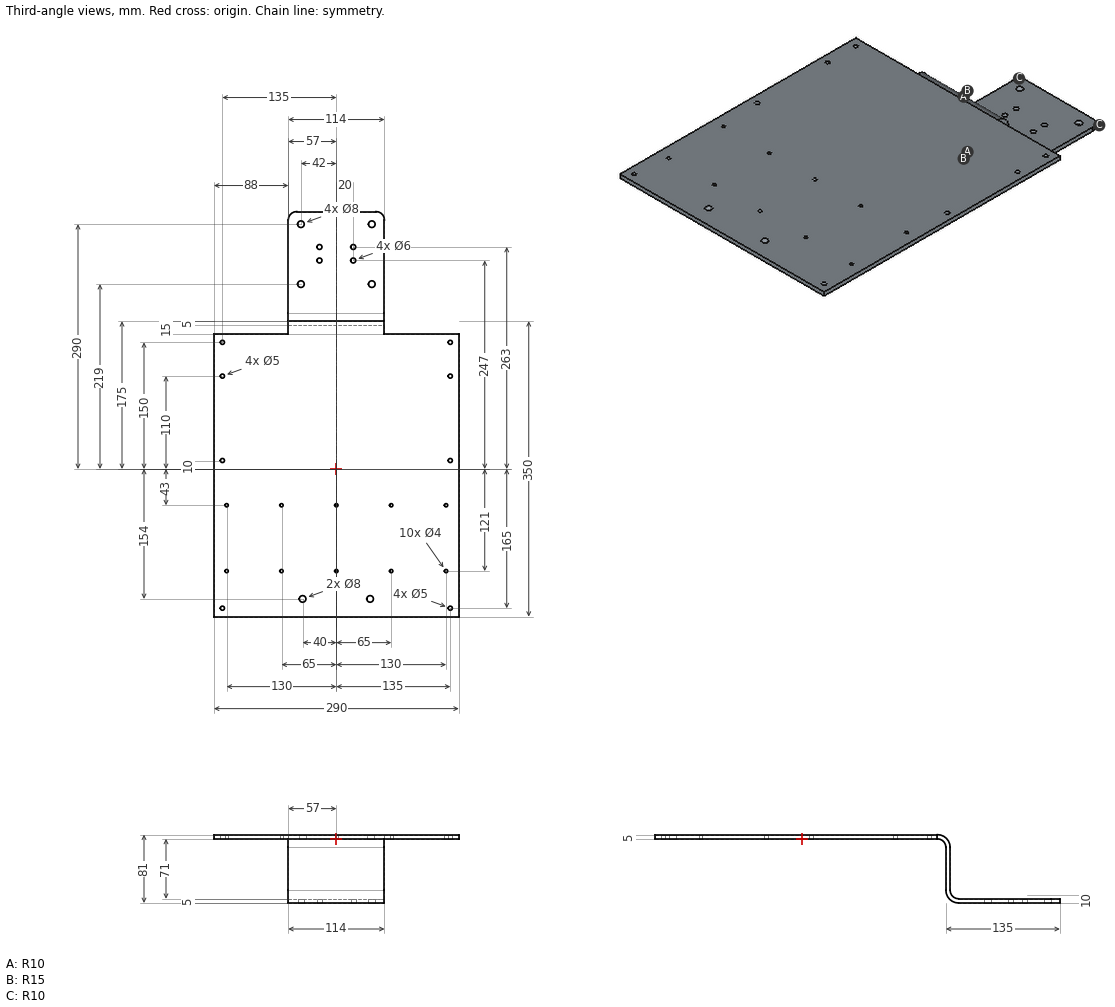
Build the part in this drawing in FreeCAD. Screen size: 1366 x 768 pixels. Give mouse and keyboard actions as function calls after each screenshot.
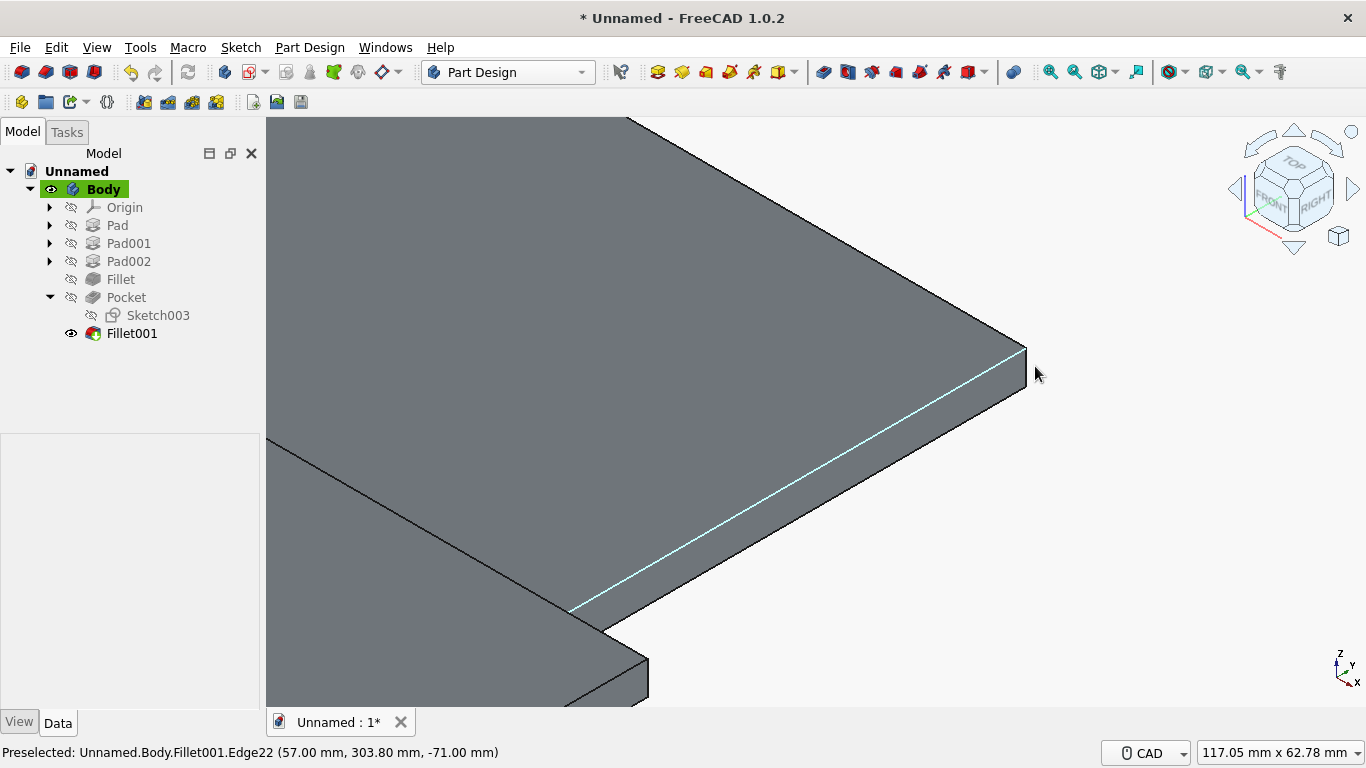
click(1052, 72)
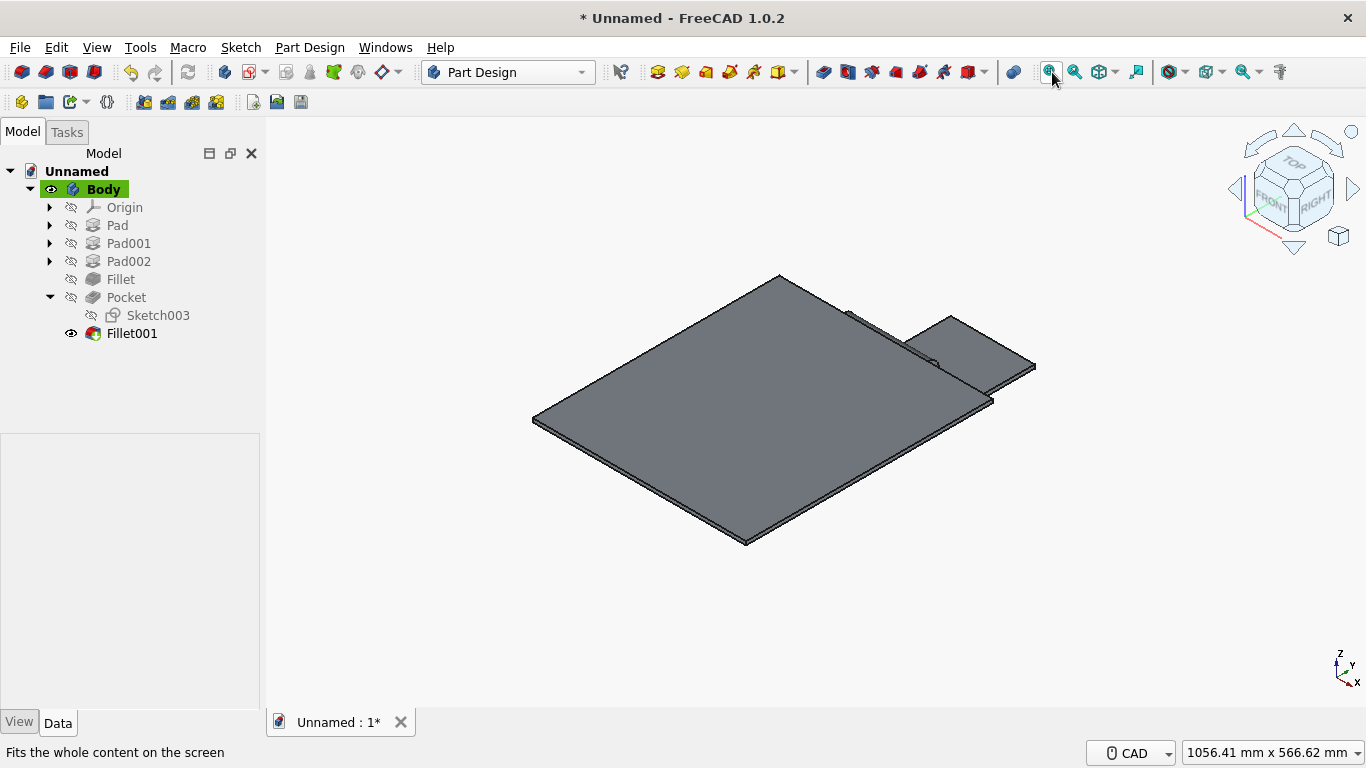
key(2)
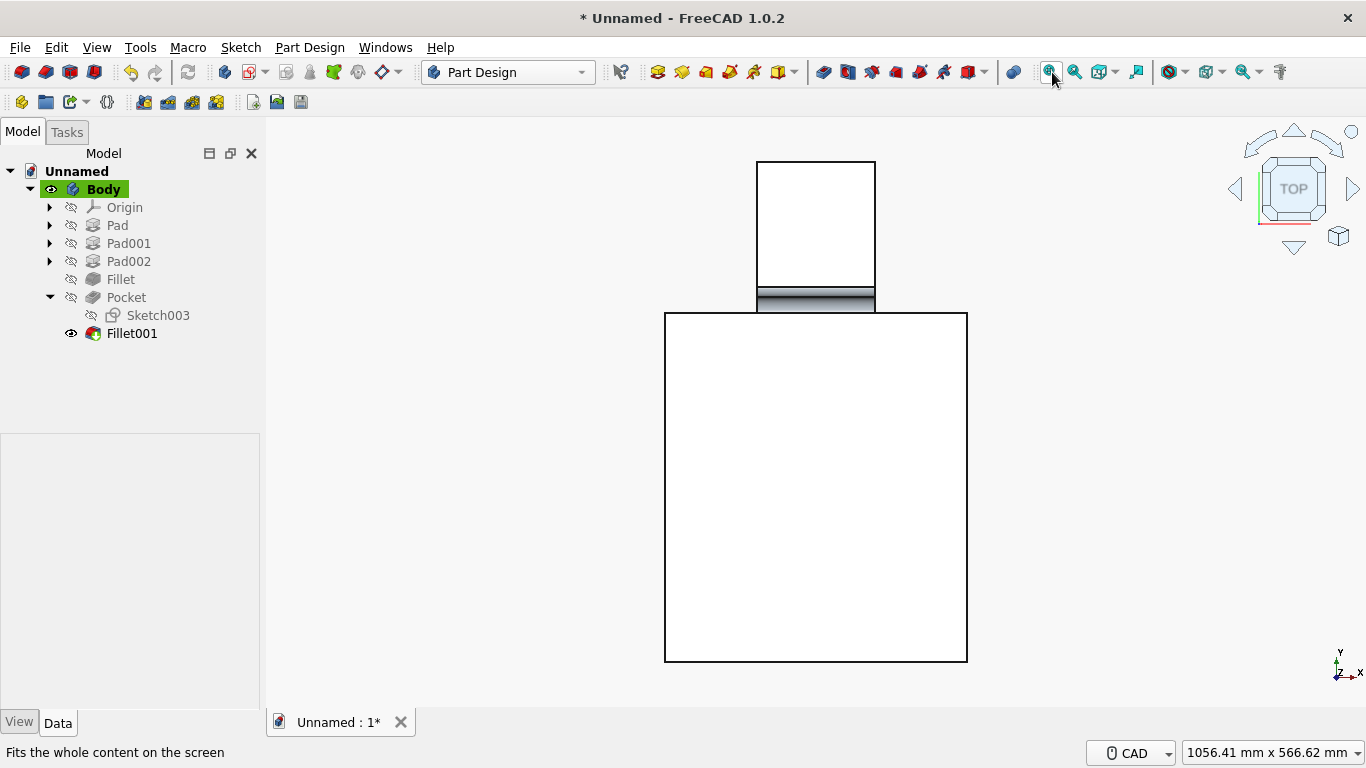
scroll(875, 161, up, 11)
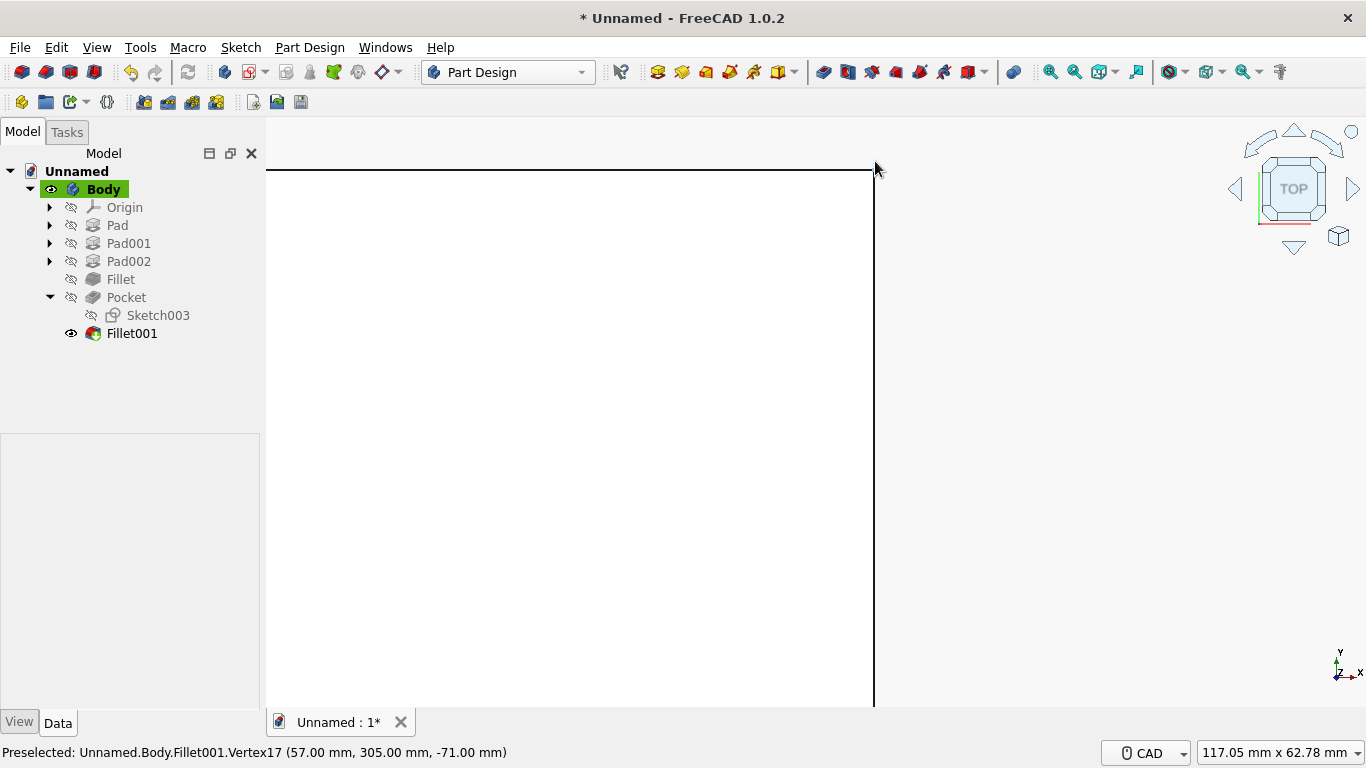
click(1052, 72)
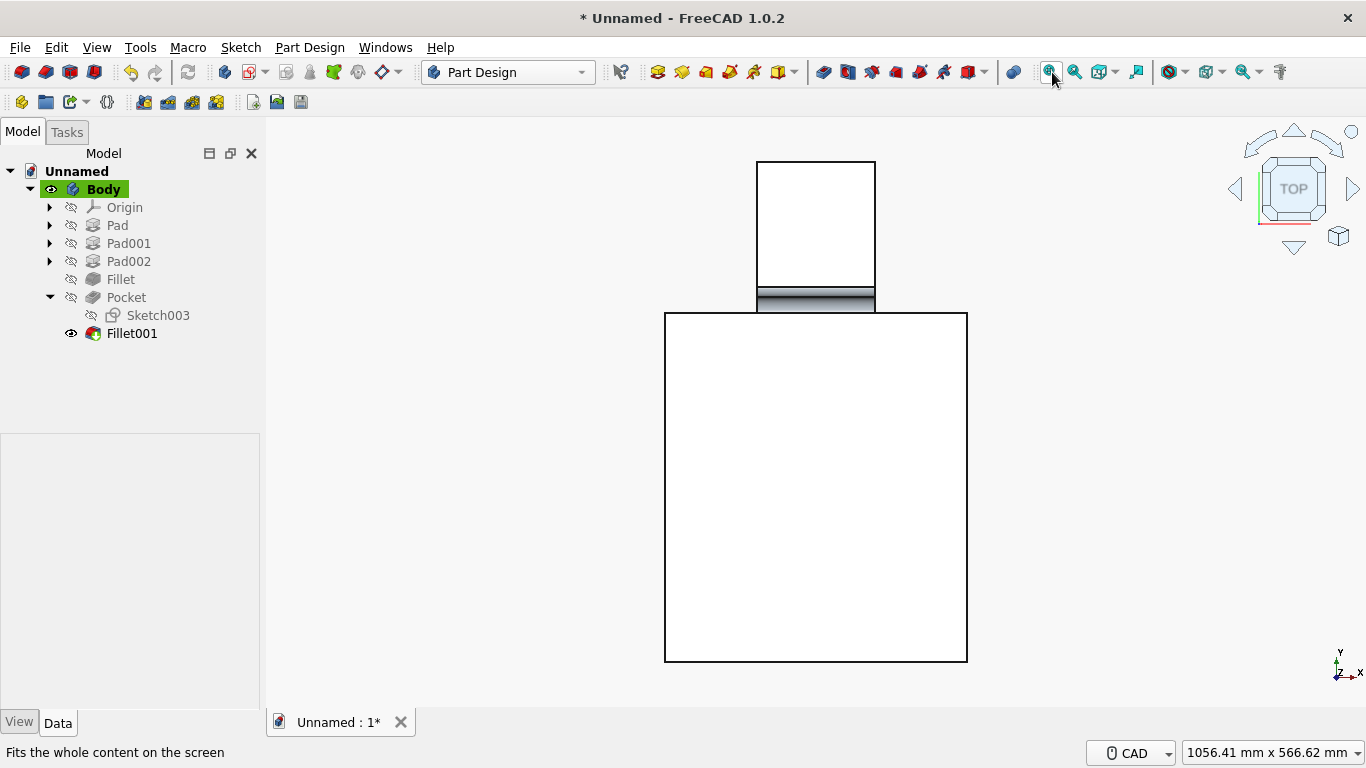
key(1)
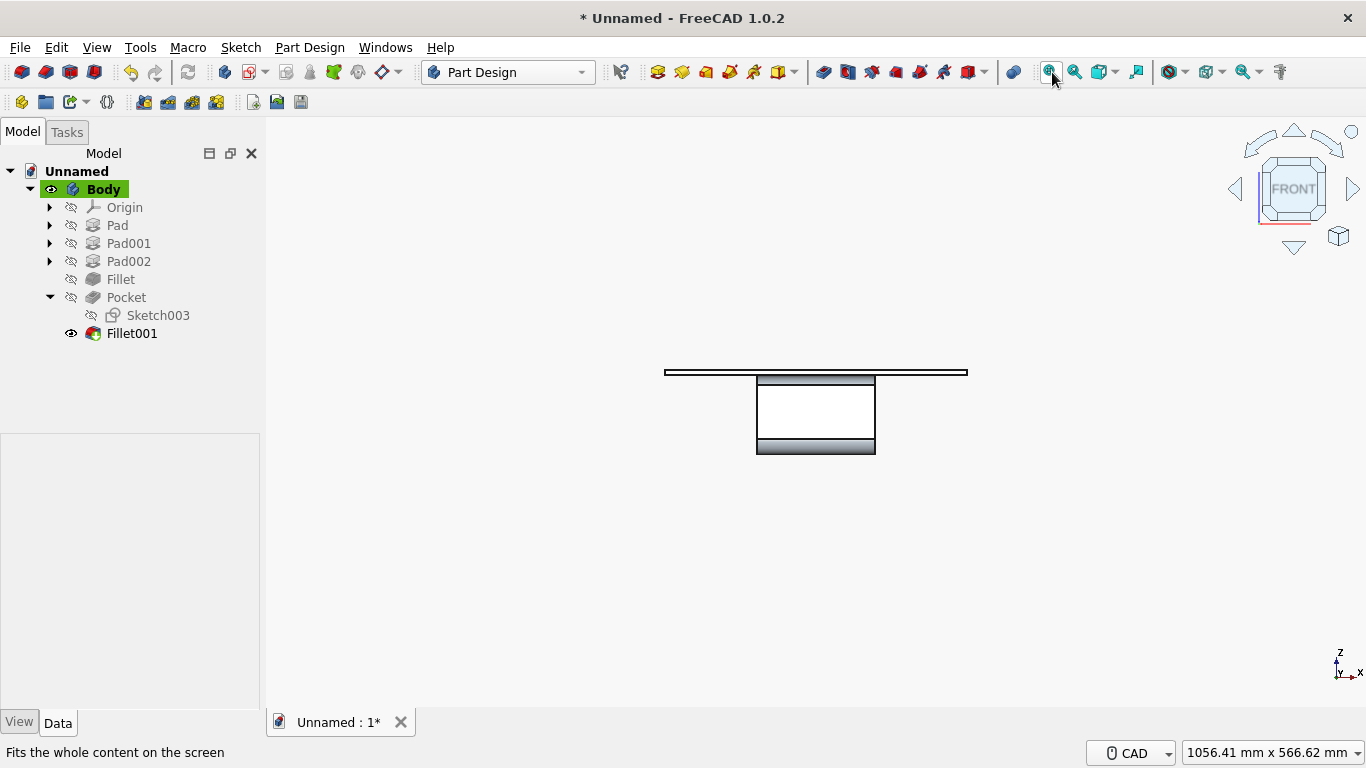
click(1052, 72)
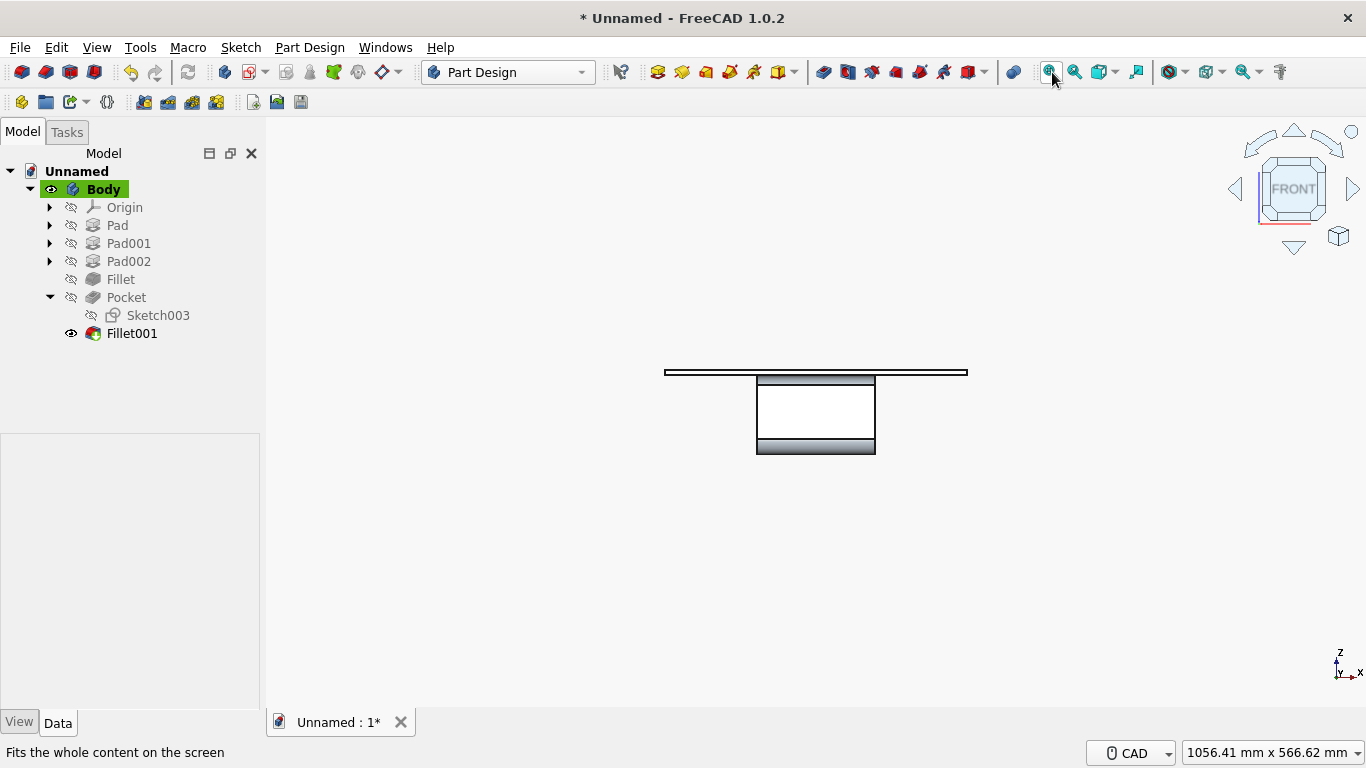
scroll(875, 451, up, 11)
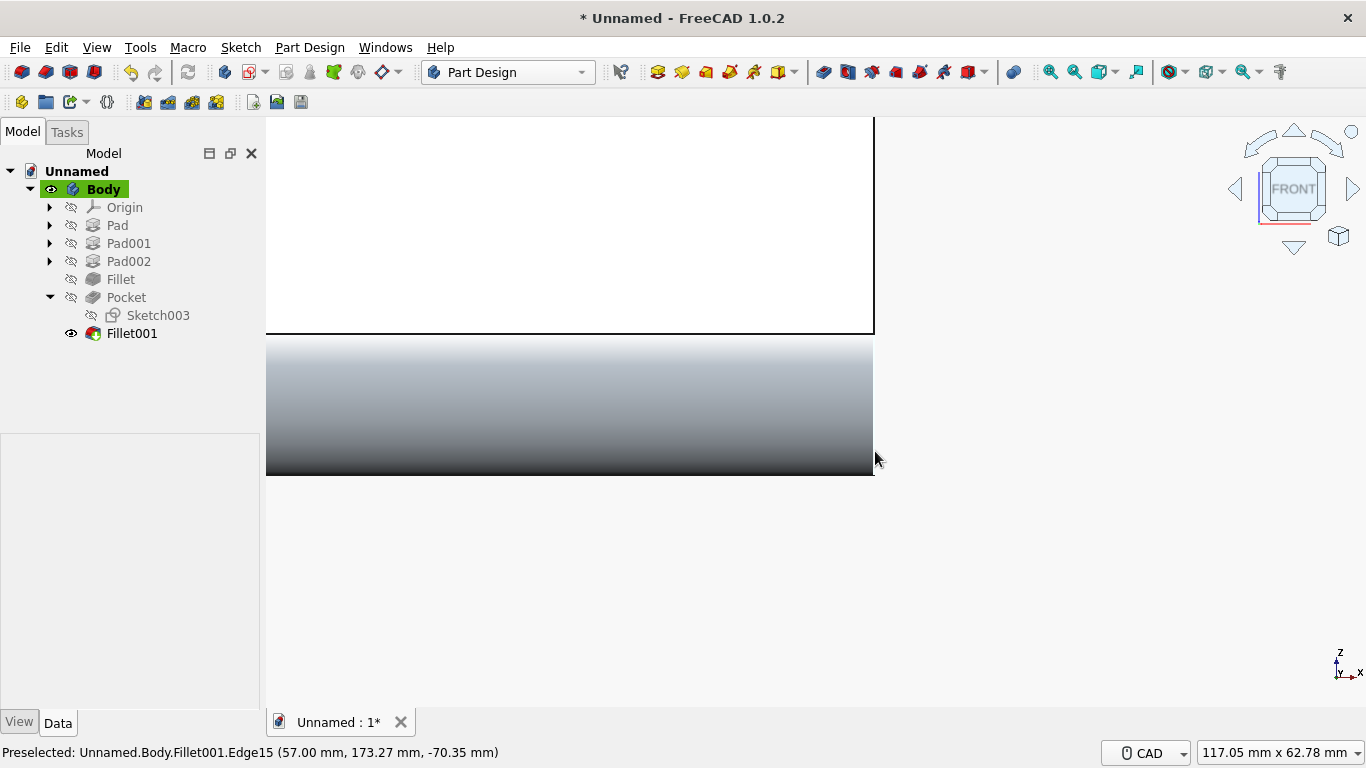
key(v)
key(f)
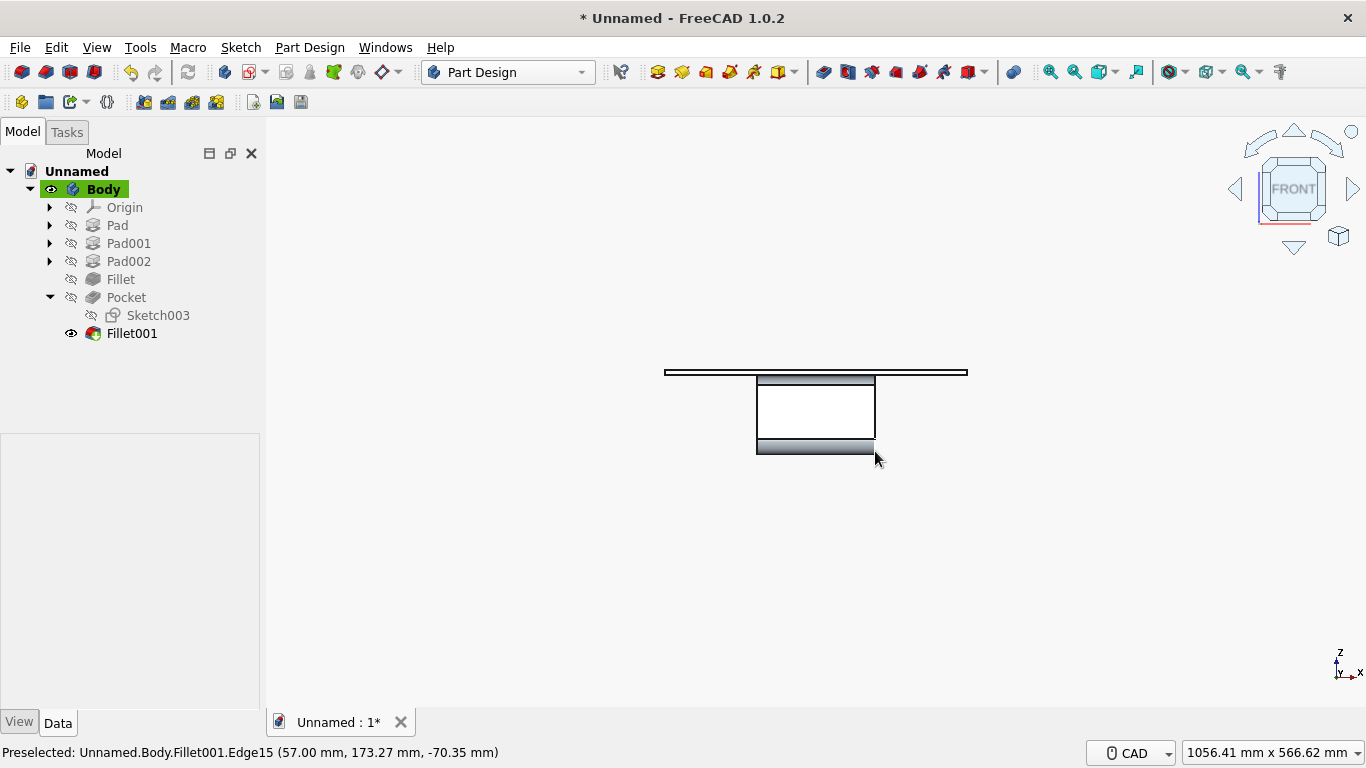
key(3)